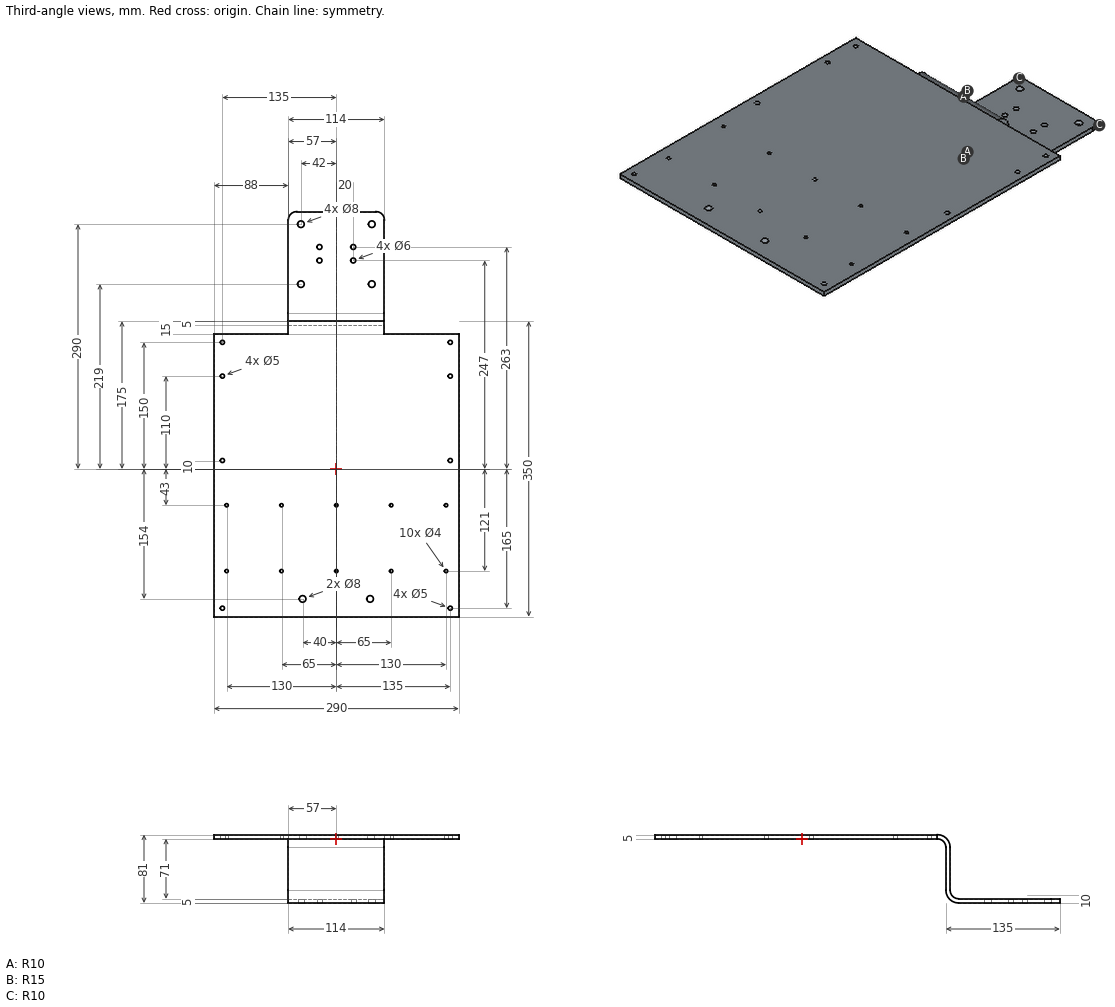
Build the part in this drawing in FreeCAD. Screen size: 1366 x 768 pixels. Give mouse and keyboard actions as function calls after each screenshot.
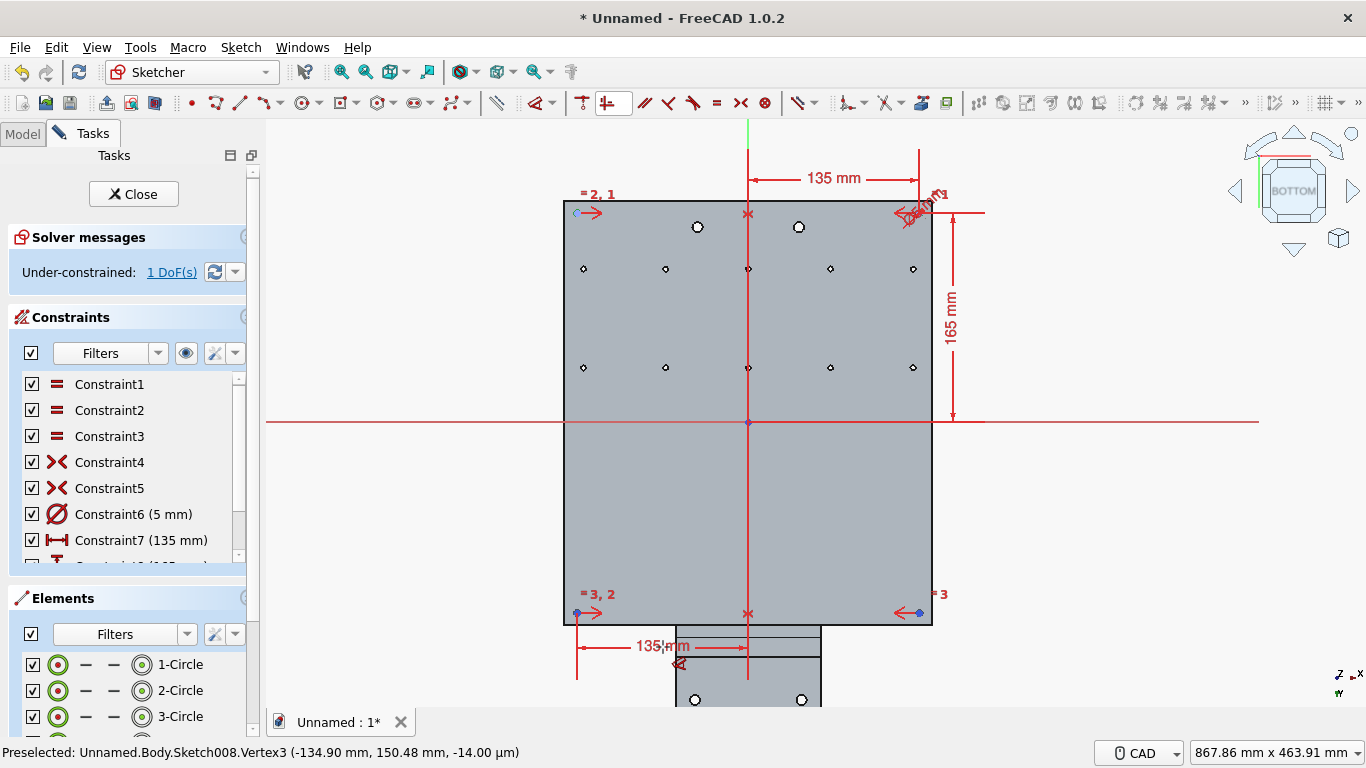
click(577, 613)
click(543, 518)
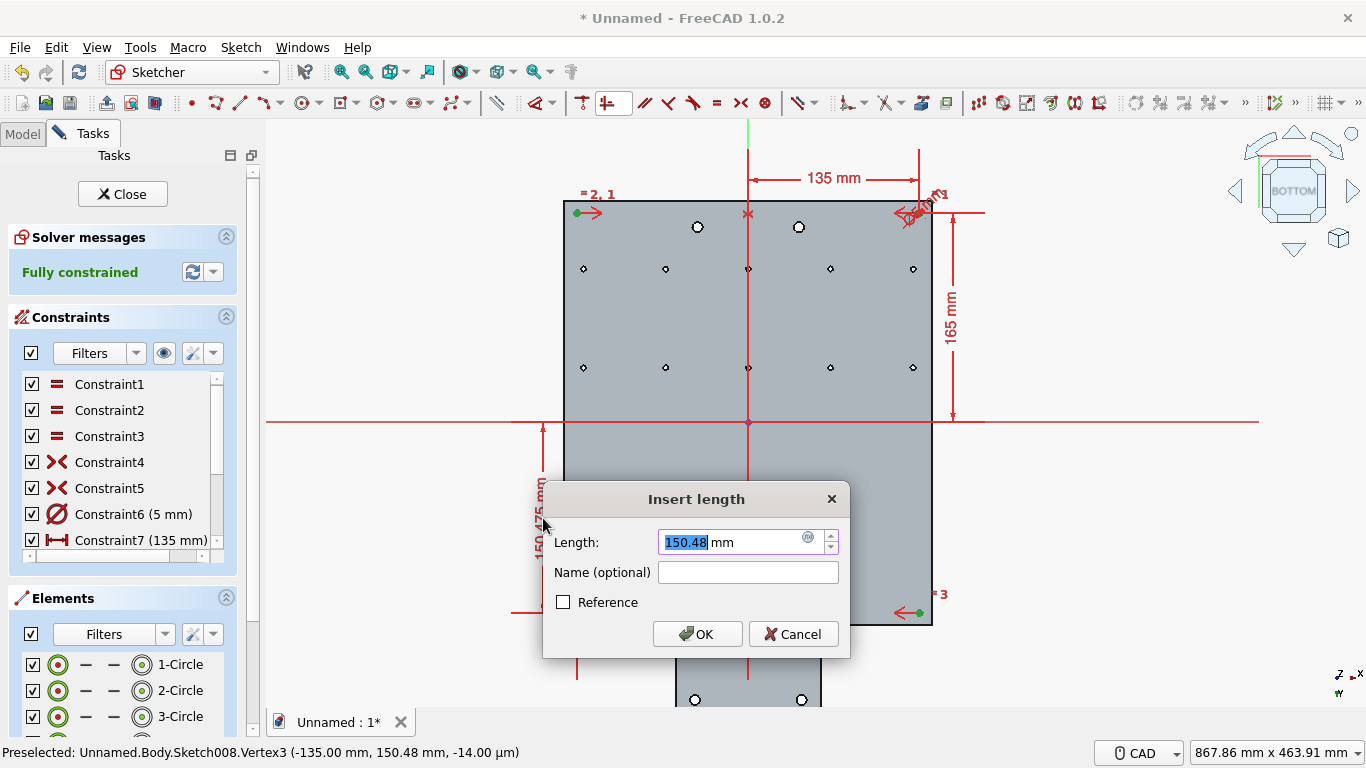
text(150)
key(Return)
key(Escape)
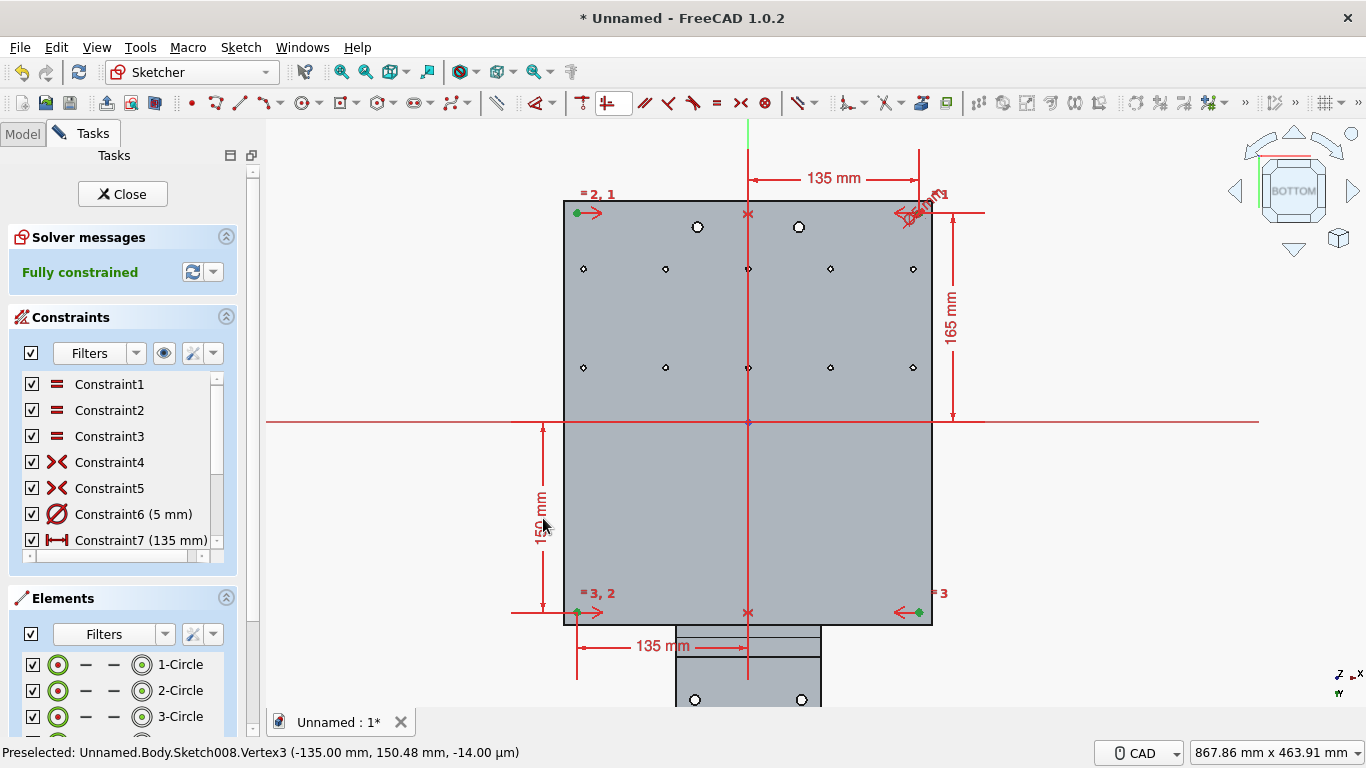
click(123, 194)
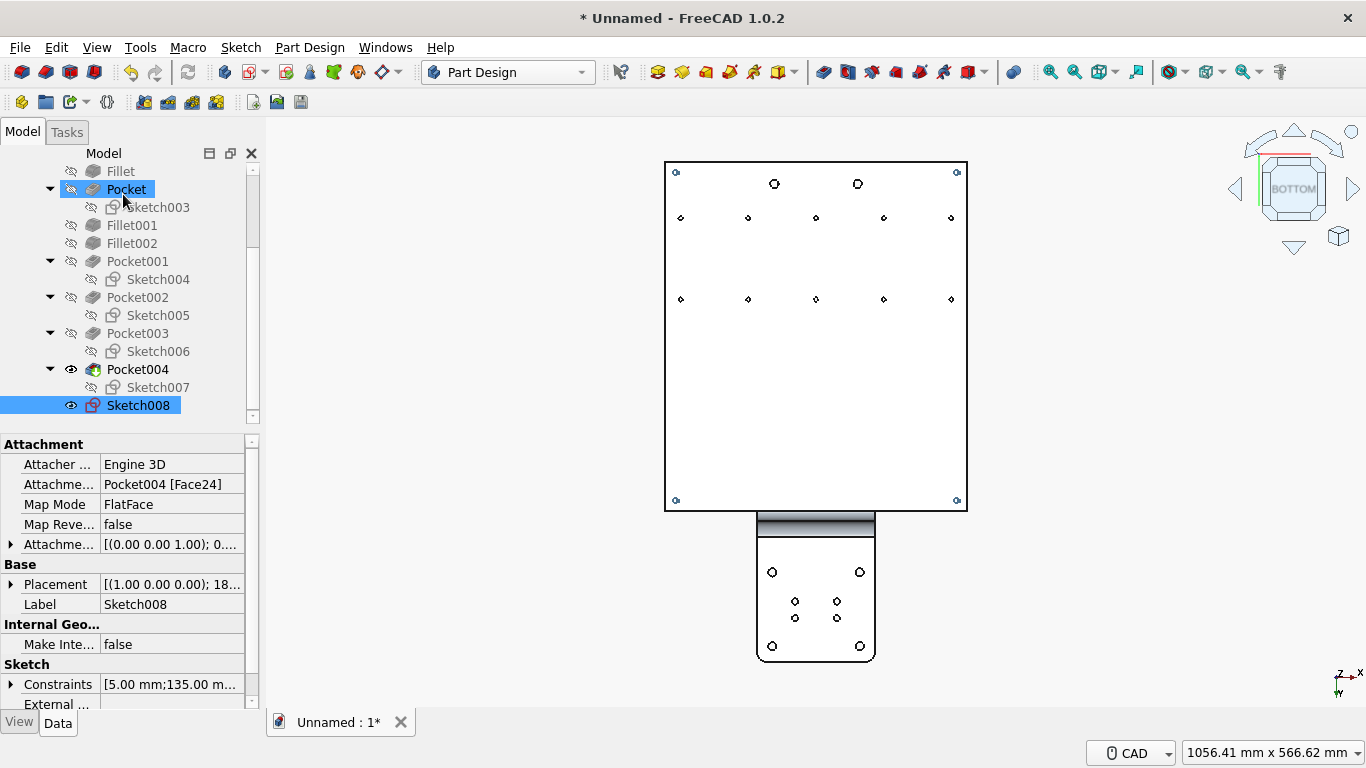
click(824, 72)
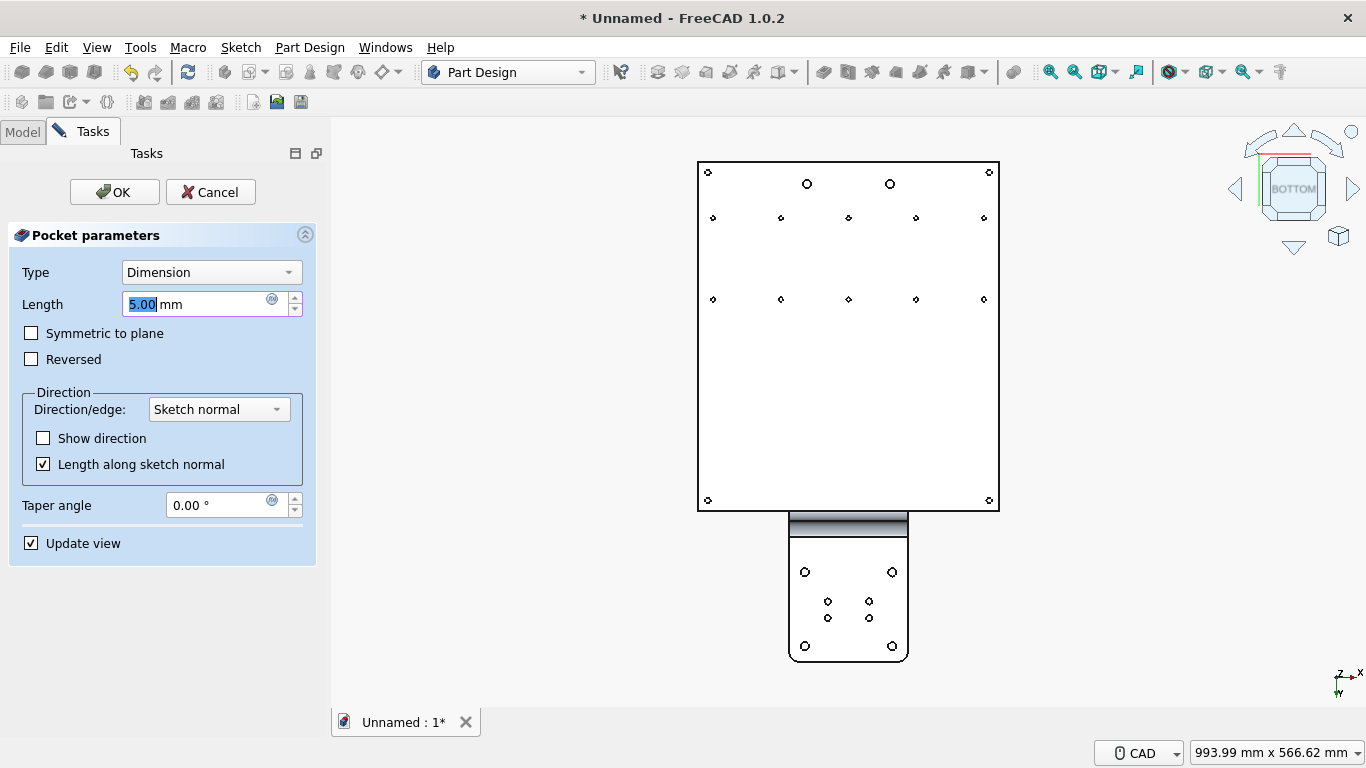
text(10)
key(Tab)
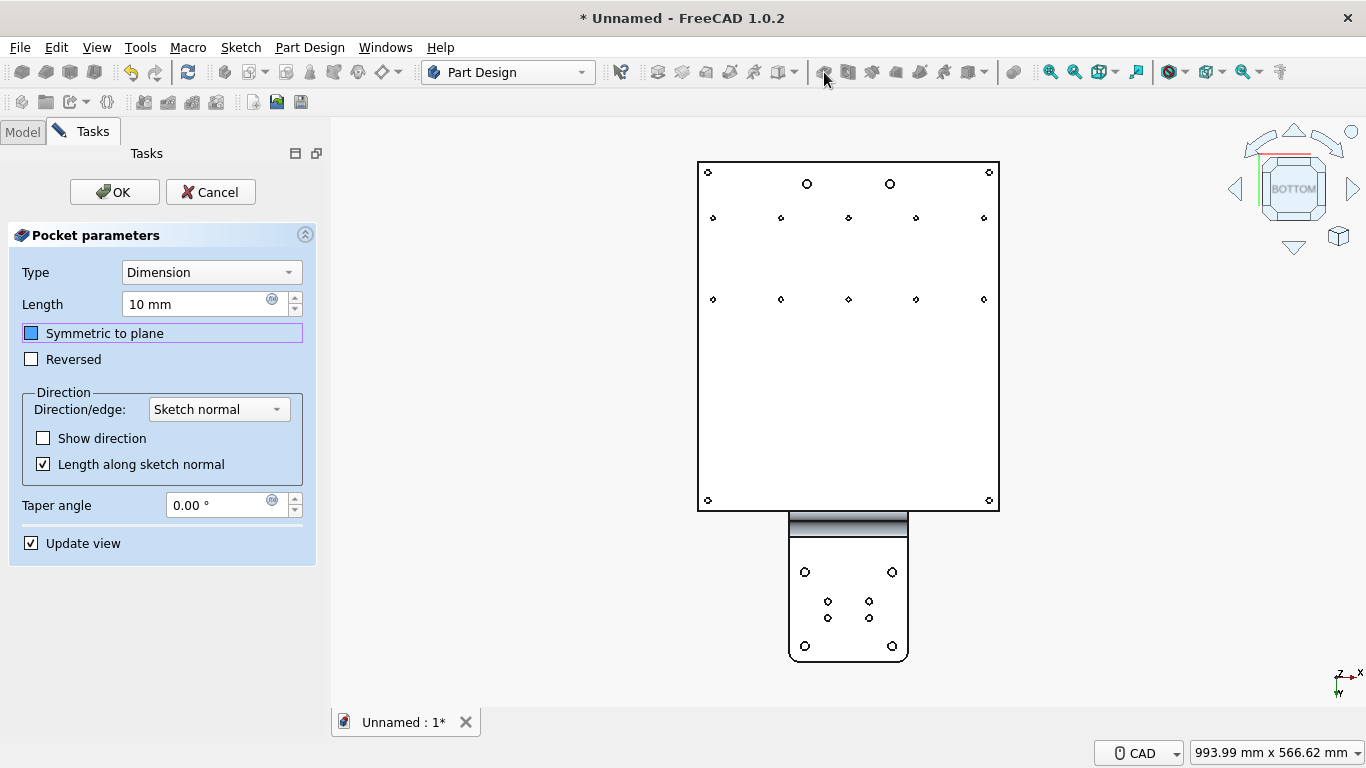
click(115, 192)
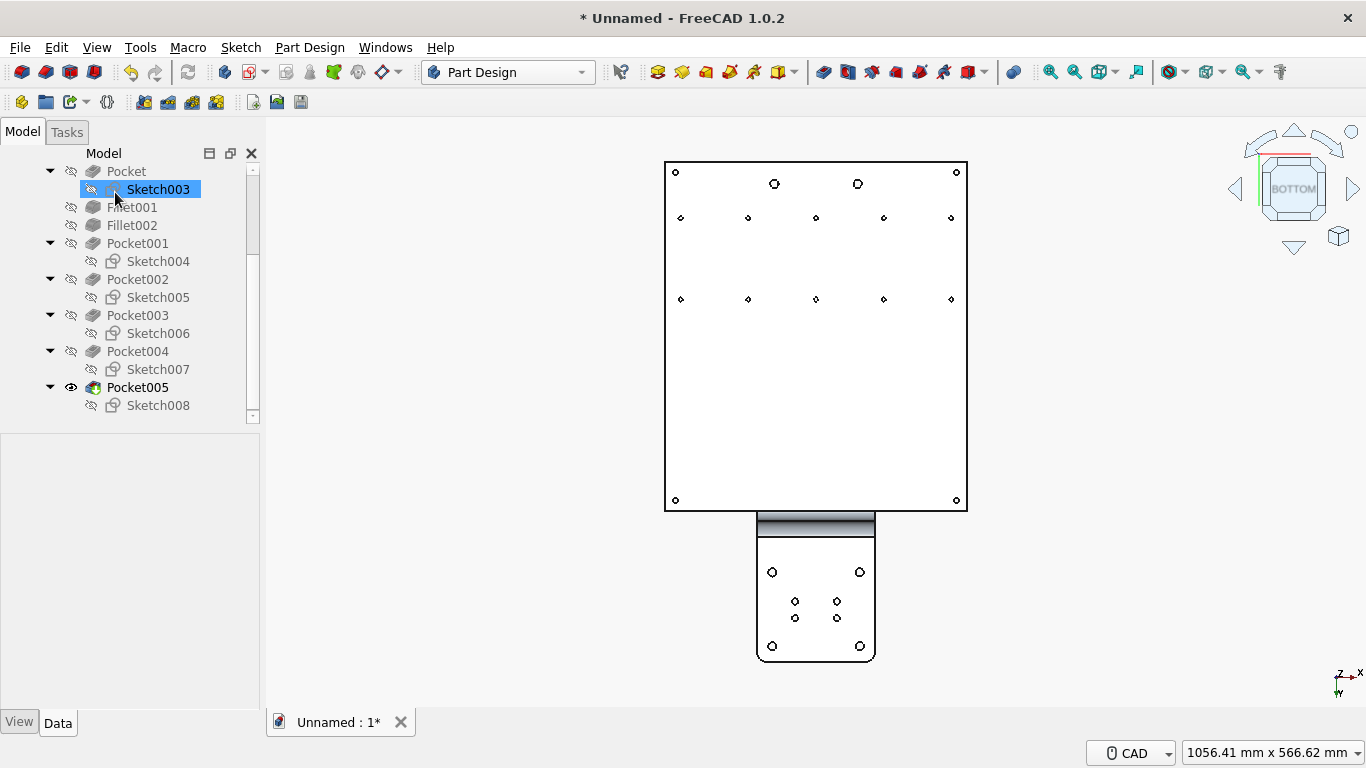
click(250, 72)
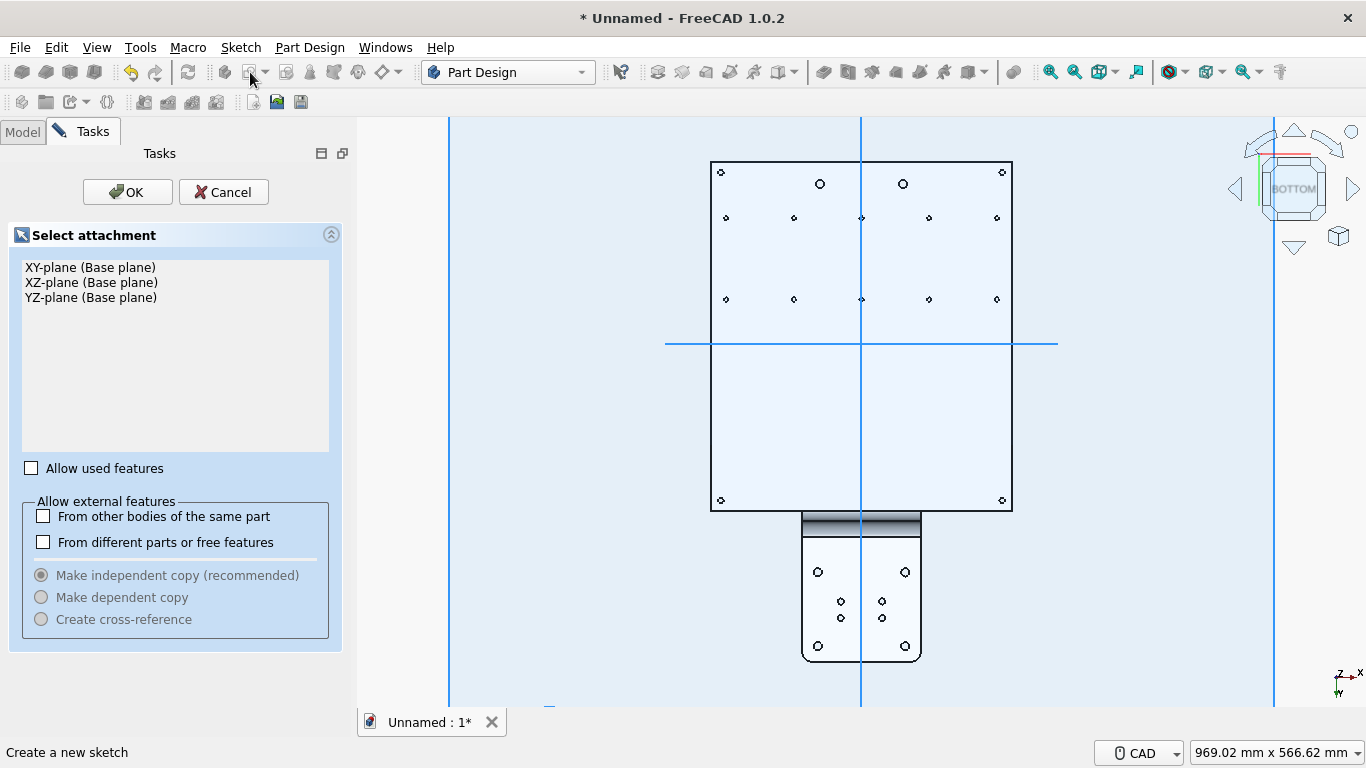
click(82, 268)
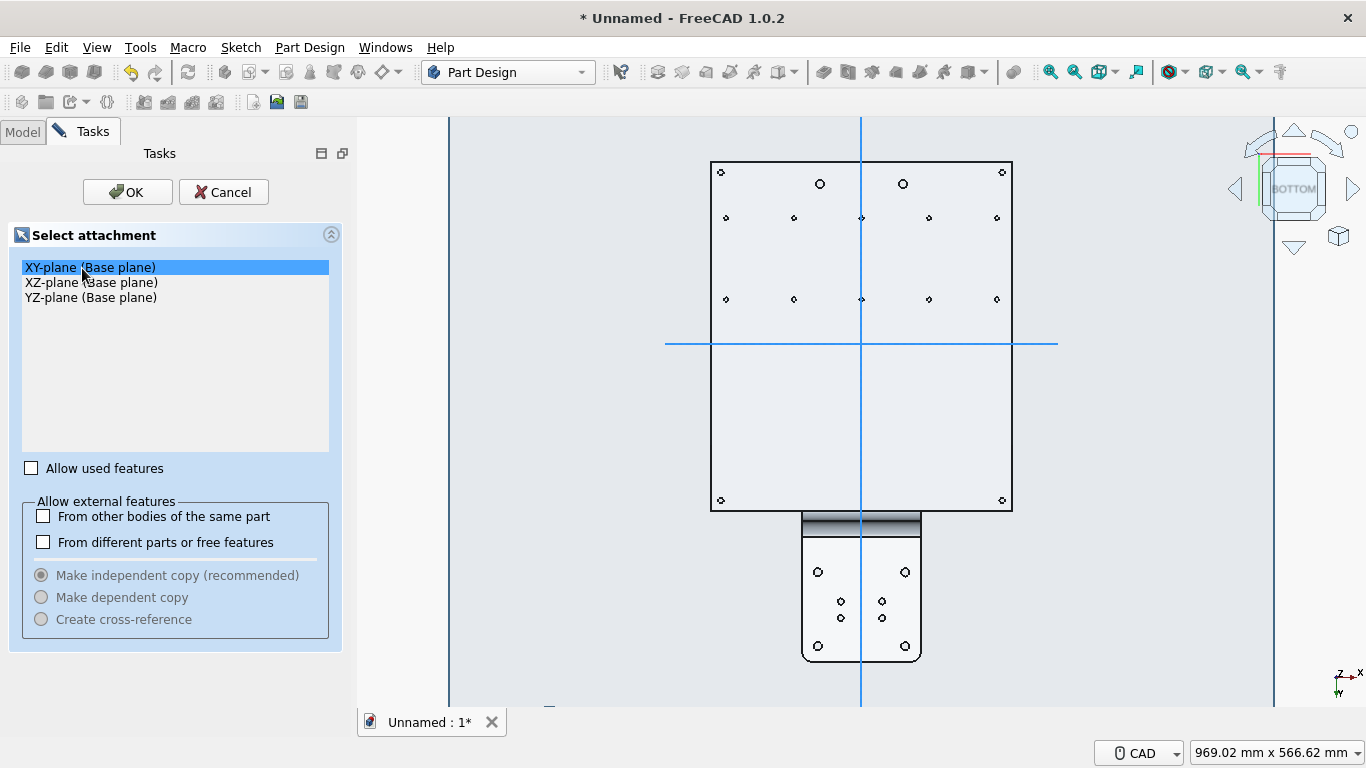
click(128, 192)